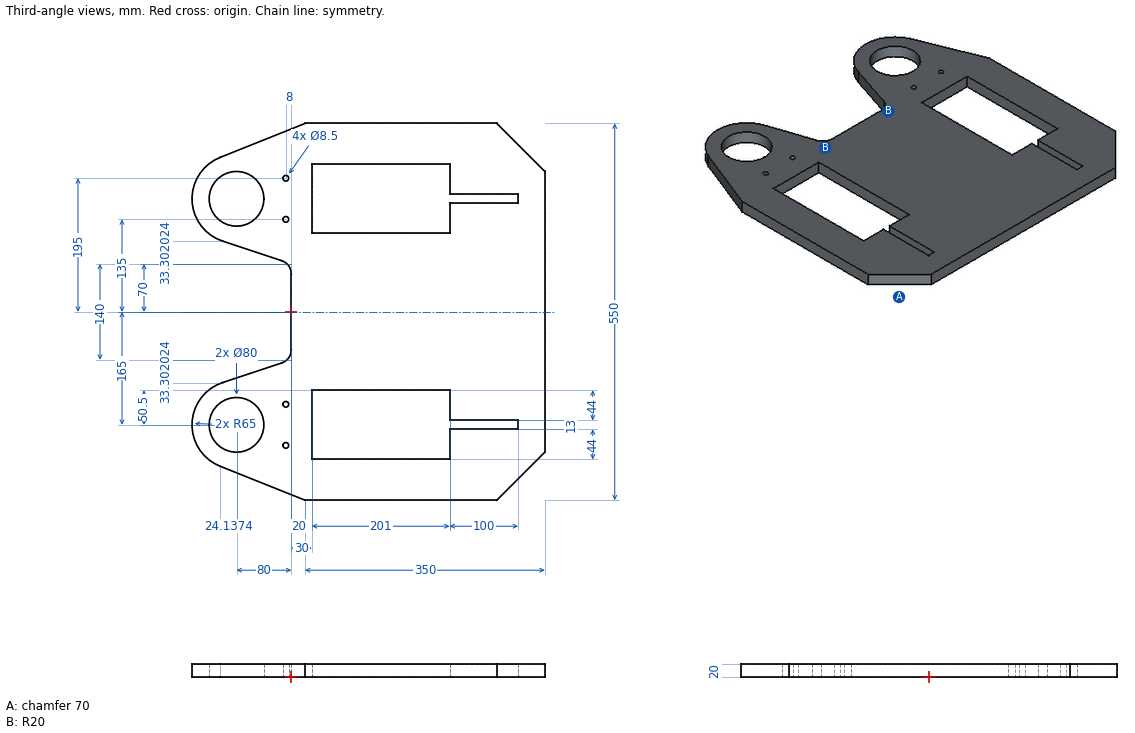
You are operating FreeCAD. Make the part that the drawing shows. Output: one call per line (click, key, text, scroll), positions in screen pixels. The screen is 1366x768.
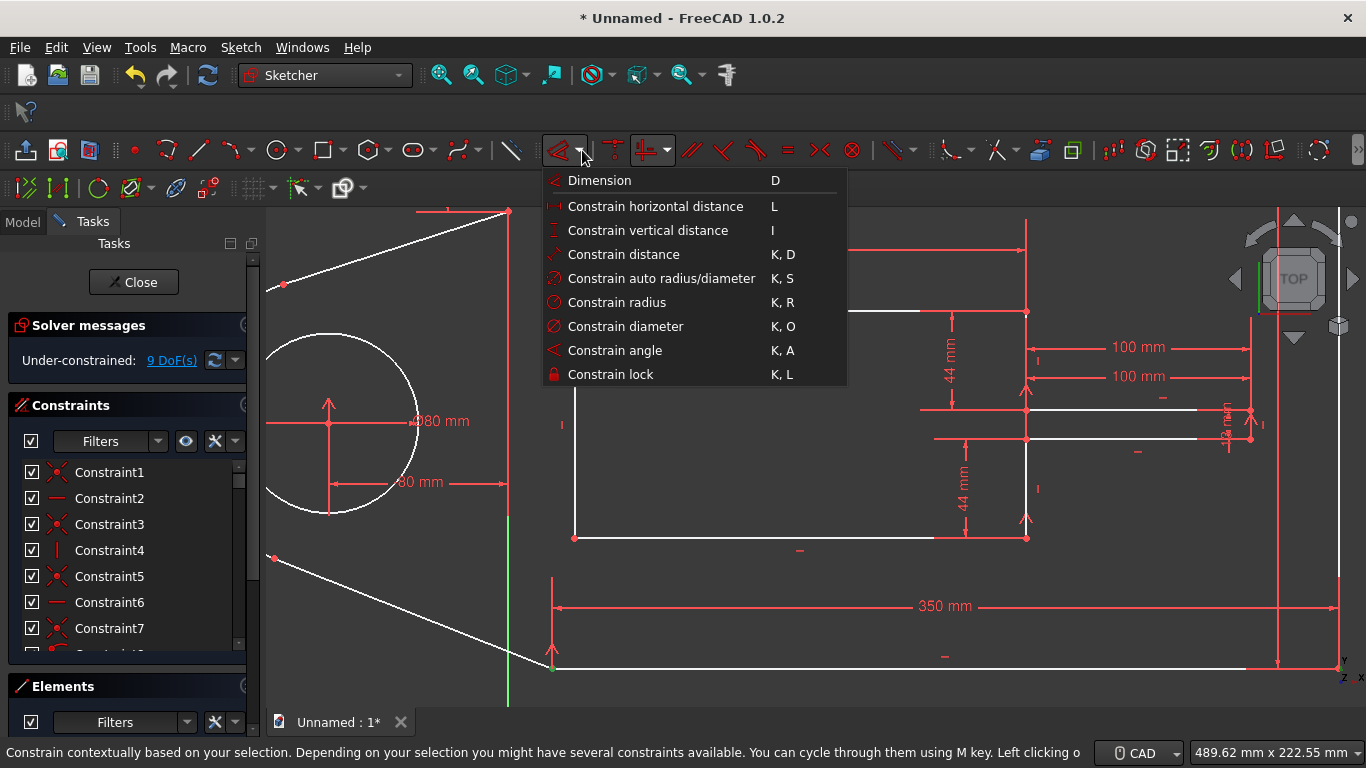
click(695, 206)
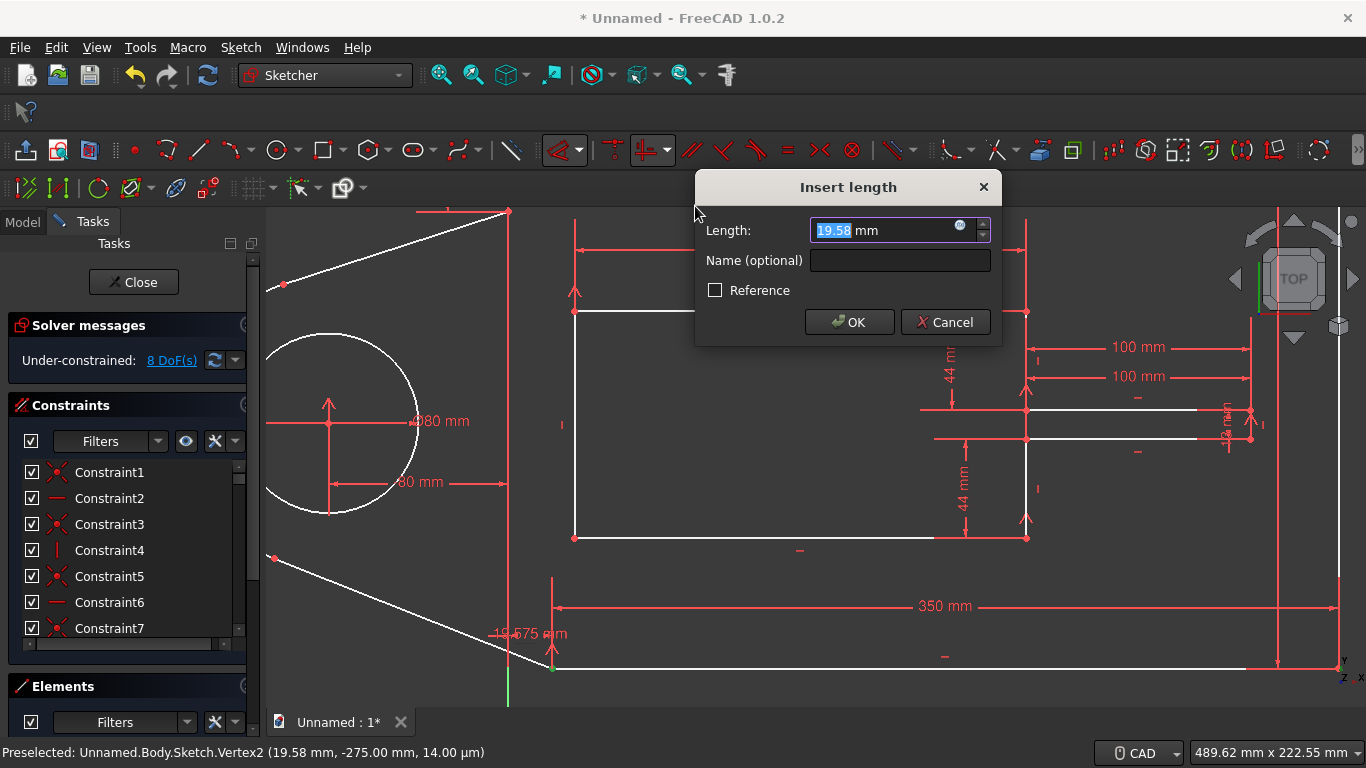
text(20)
key(Return)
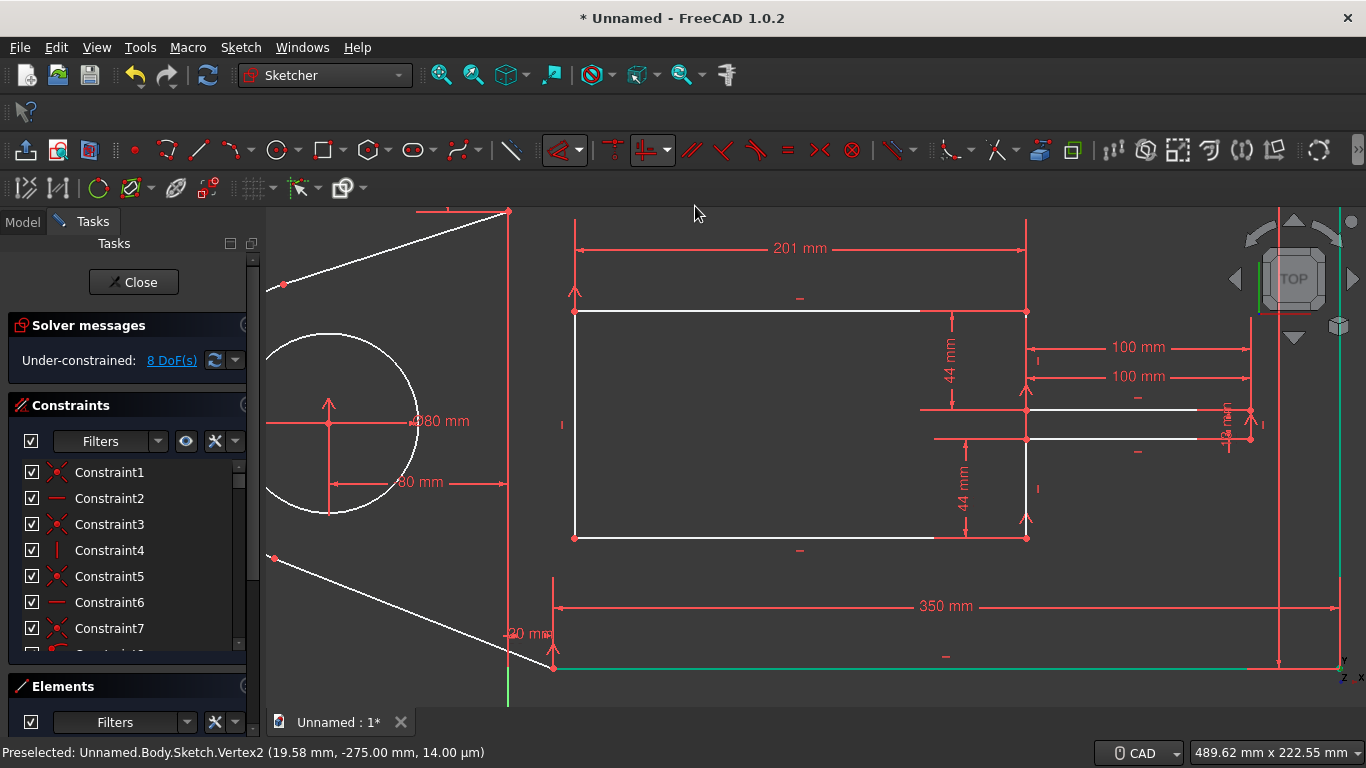
scroll(743, 590, down, 7)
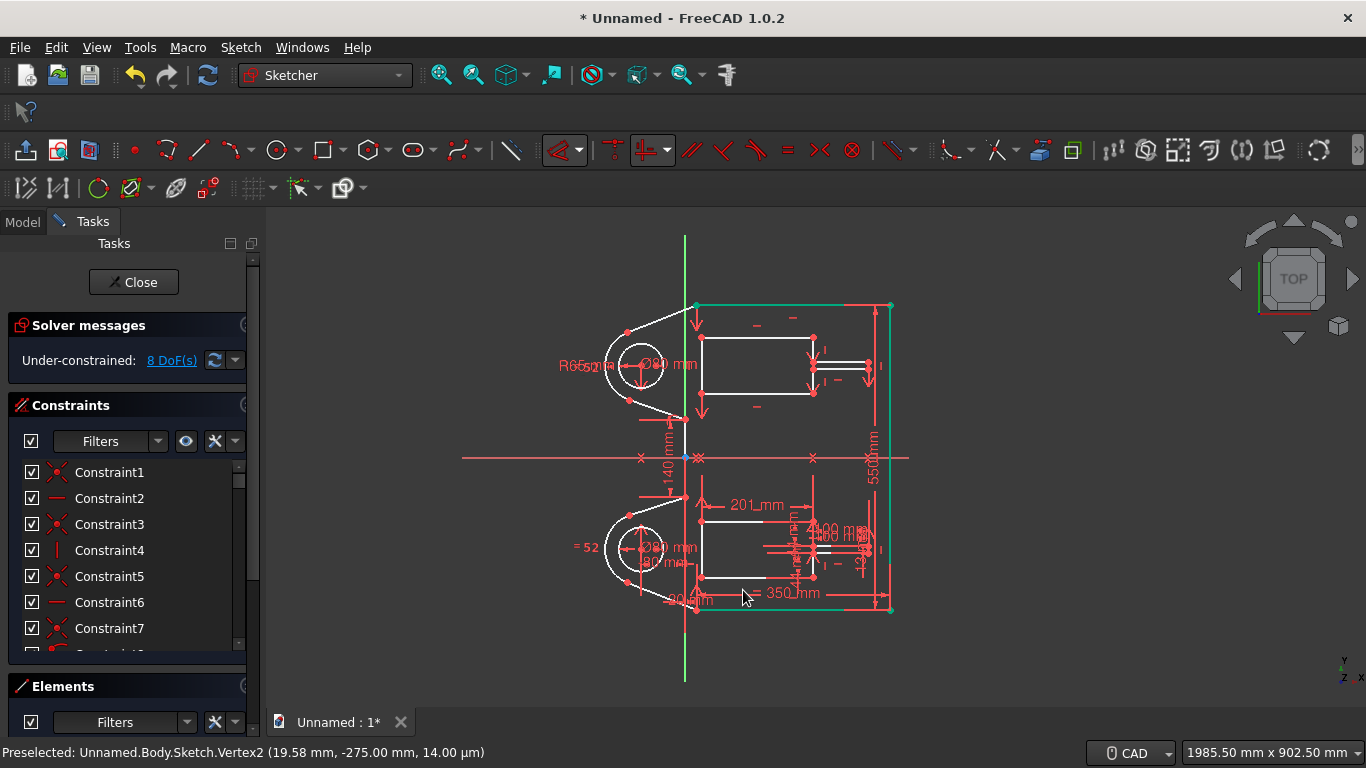
click(685, 420)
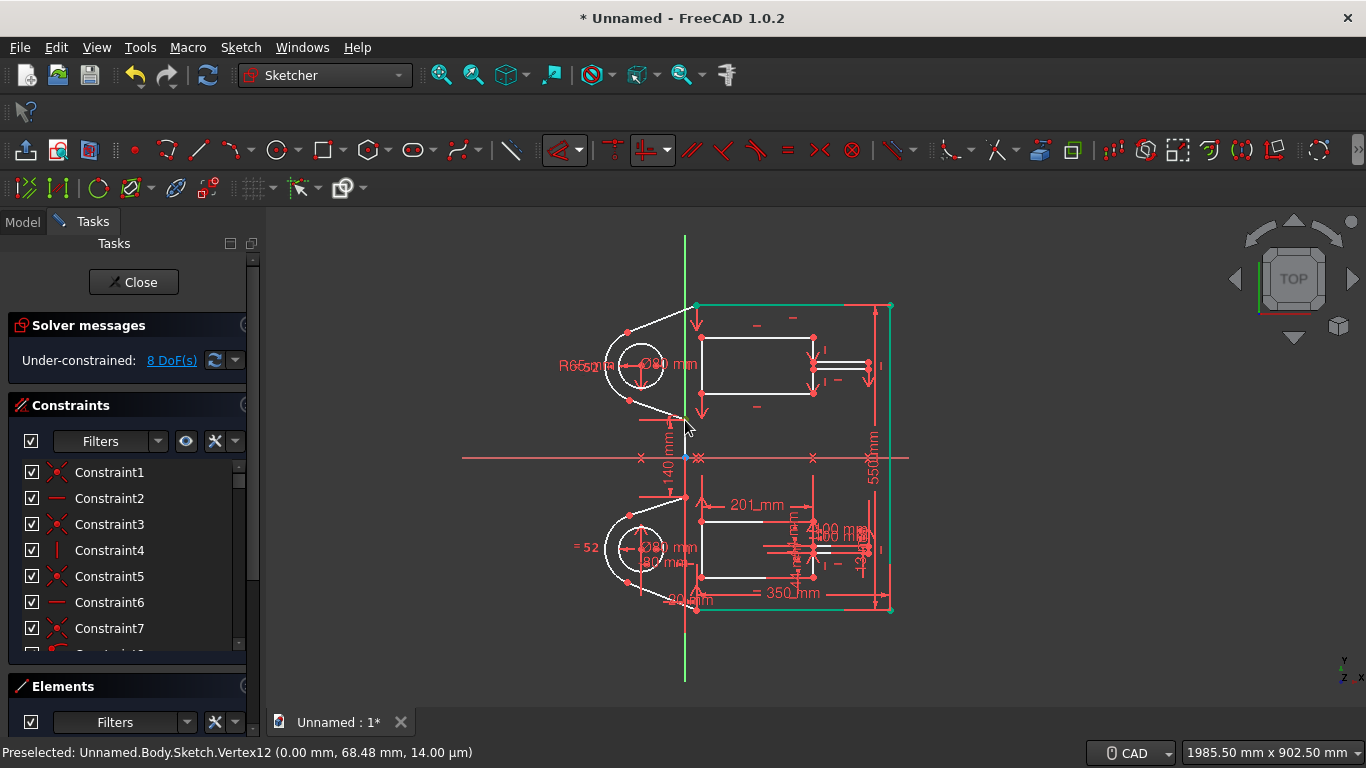
key(i)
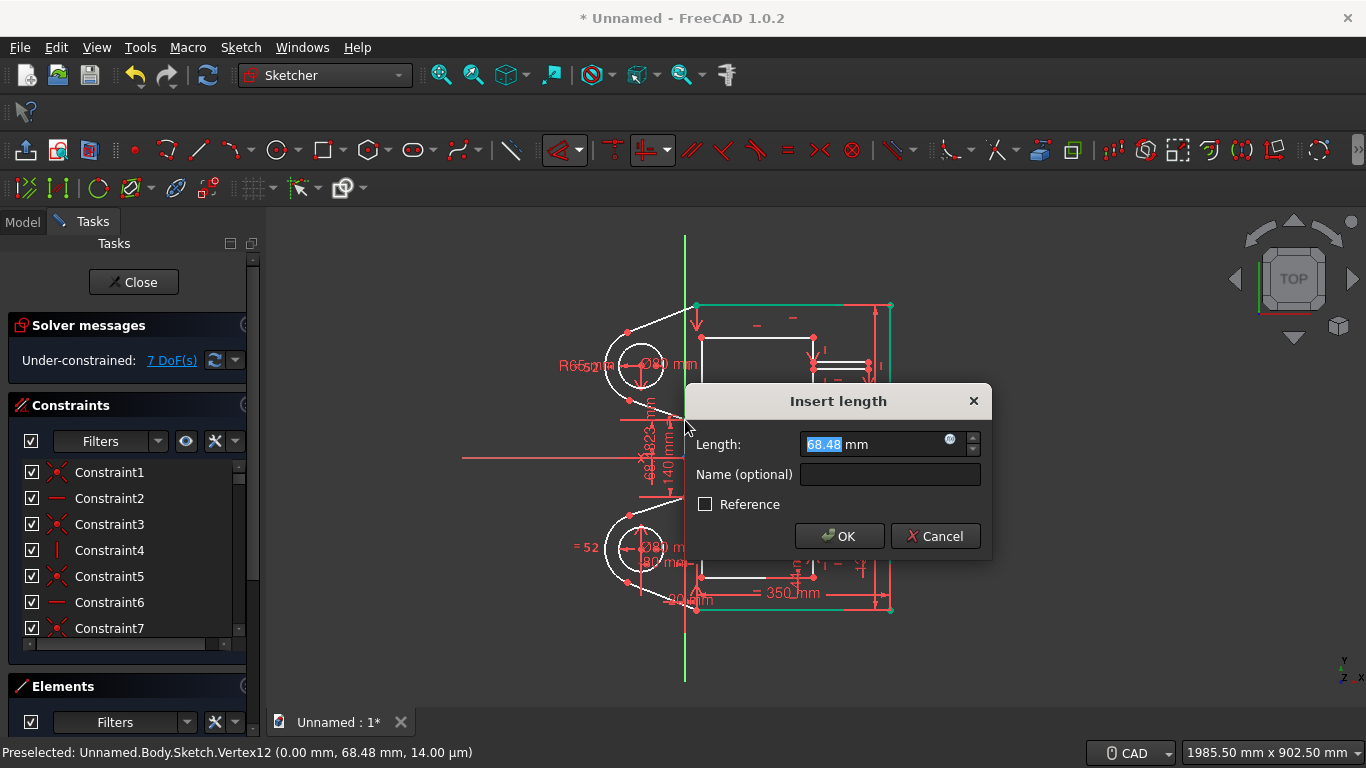
text(70)
key(Return)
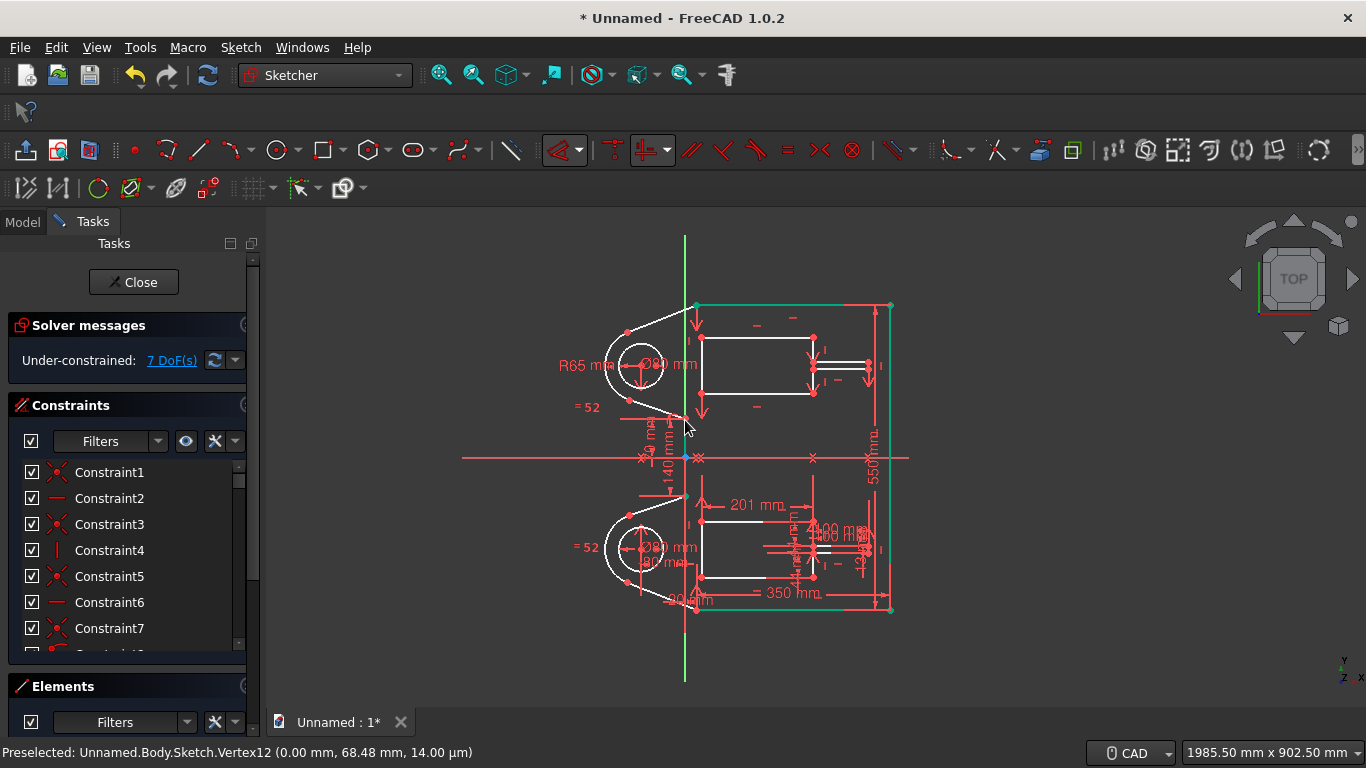
scroll(702, 522, up, 5)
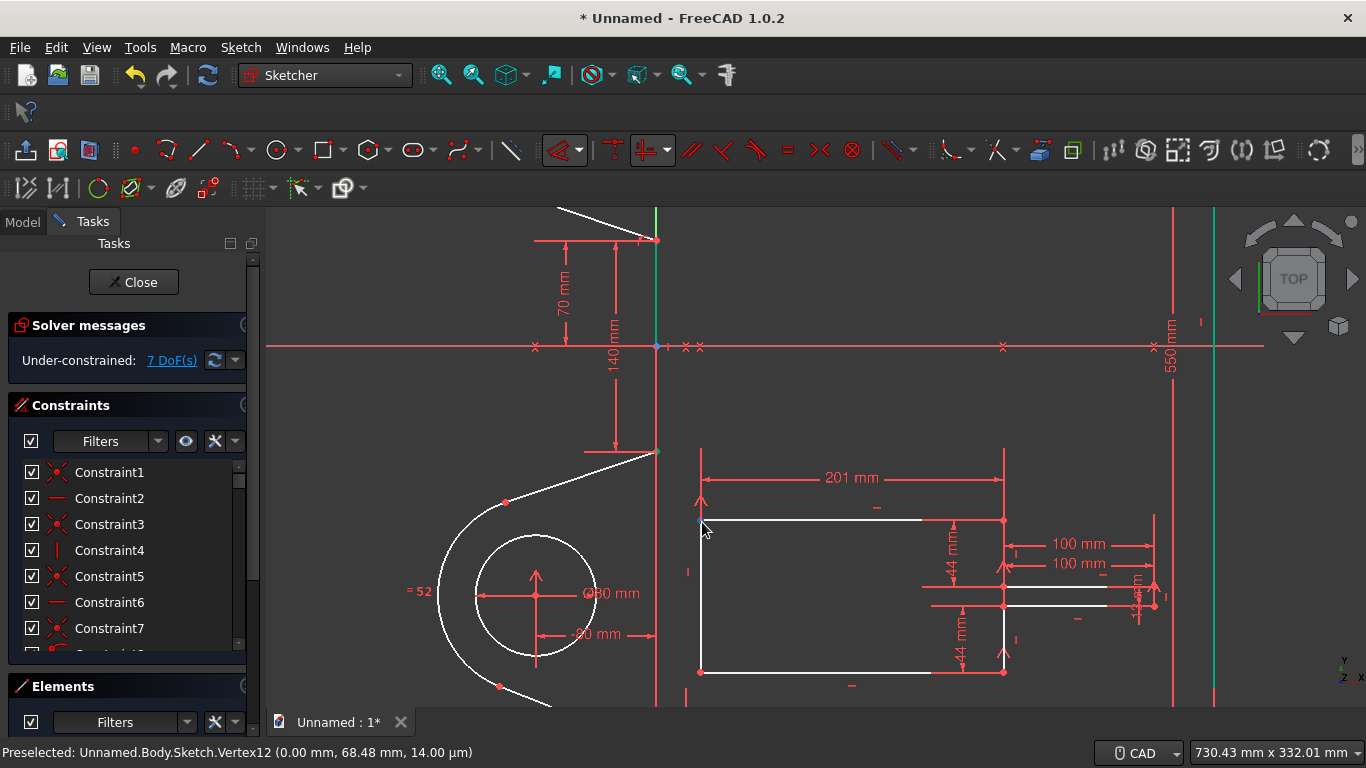
click(701, 520)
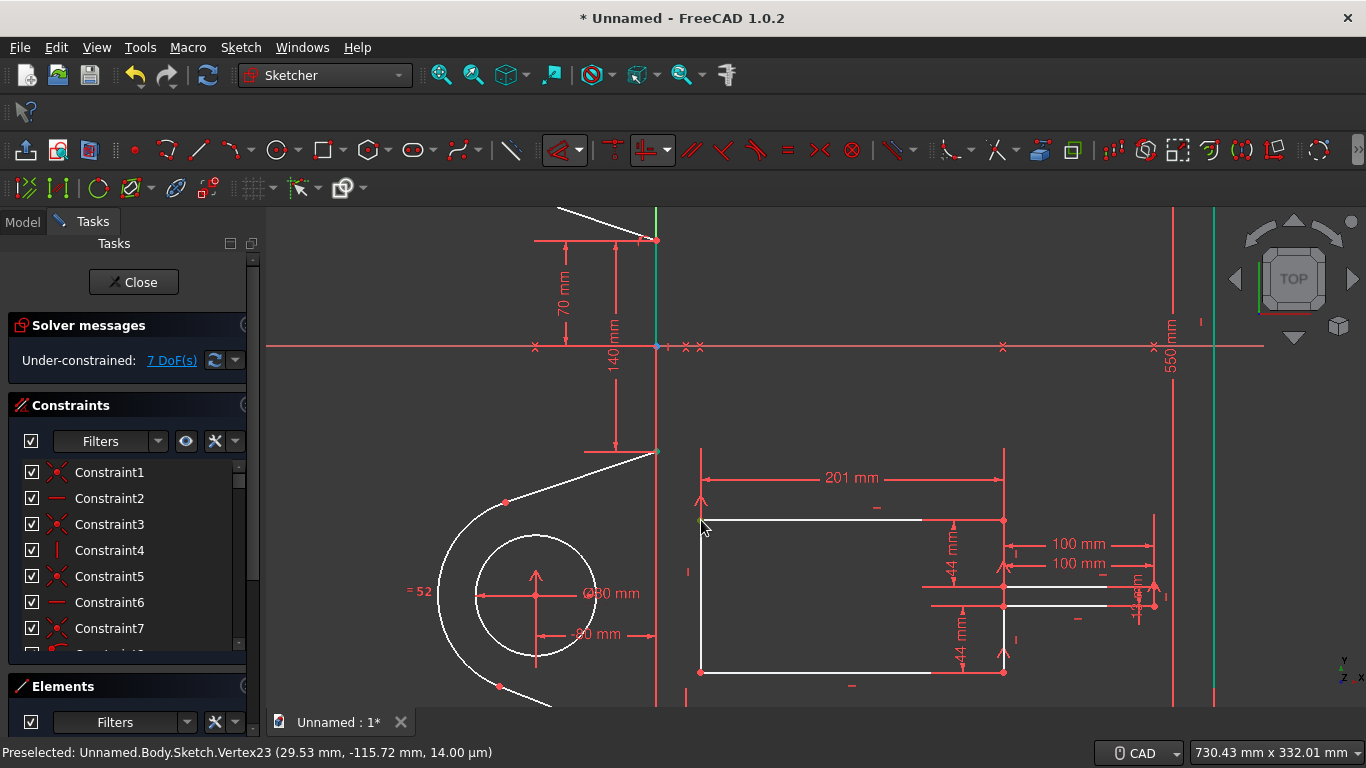
key(l)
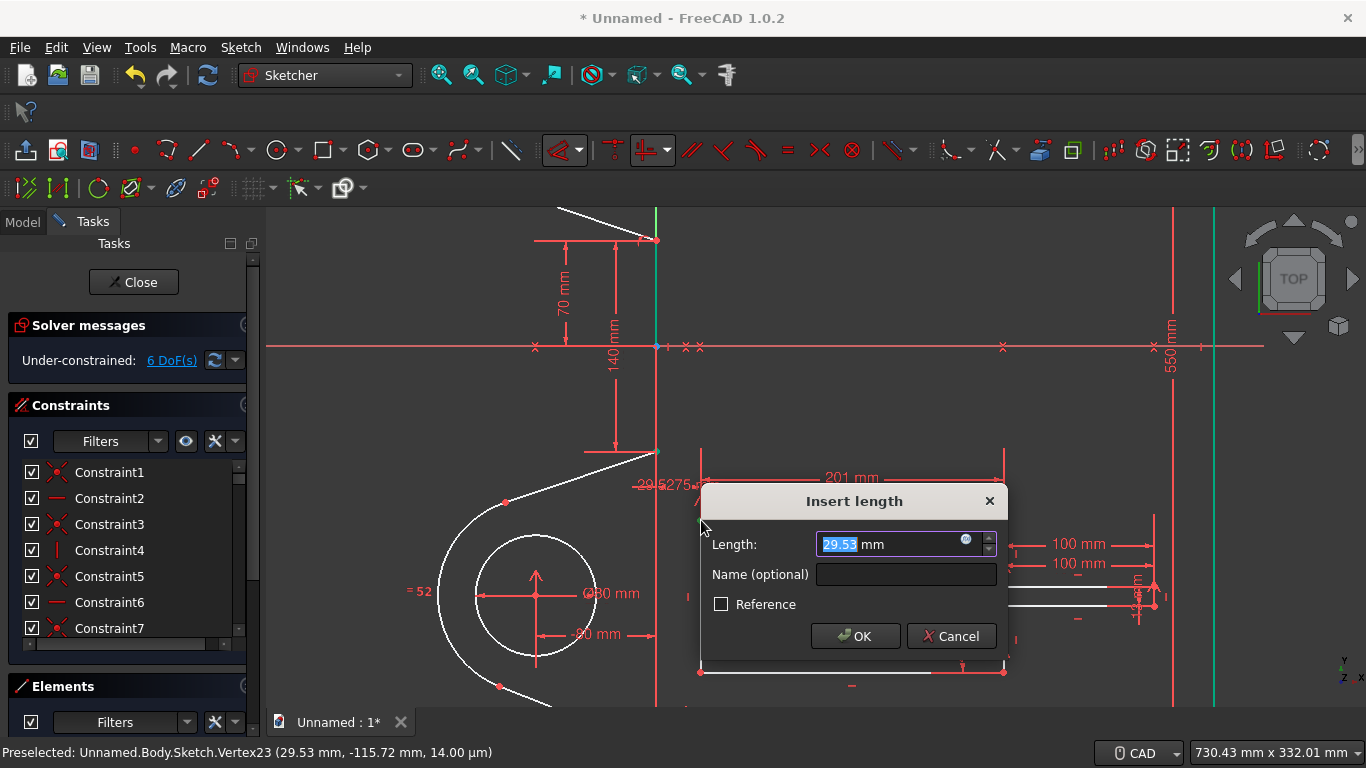
text(30)
key(Return)